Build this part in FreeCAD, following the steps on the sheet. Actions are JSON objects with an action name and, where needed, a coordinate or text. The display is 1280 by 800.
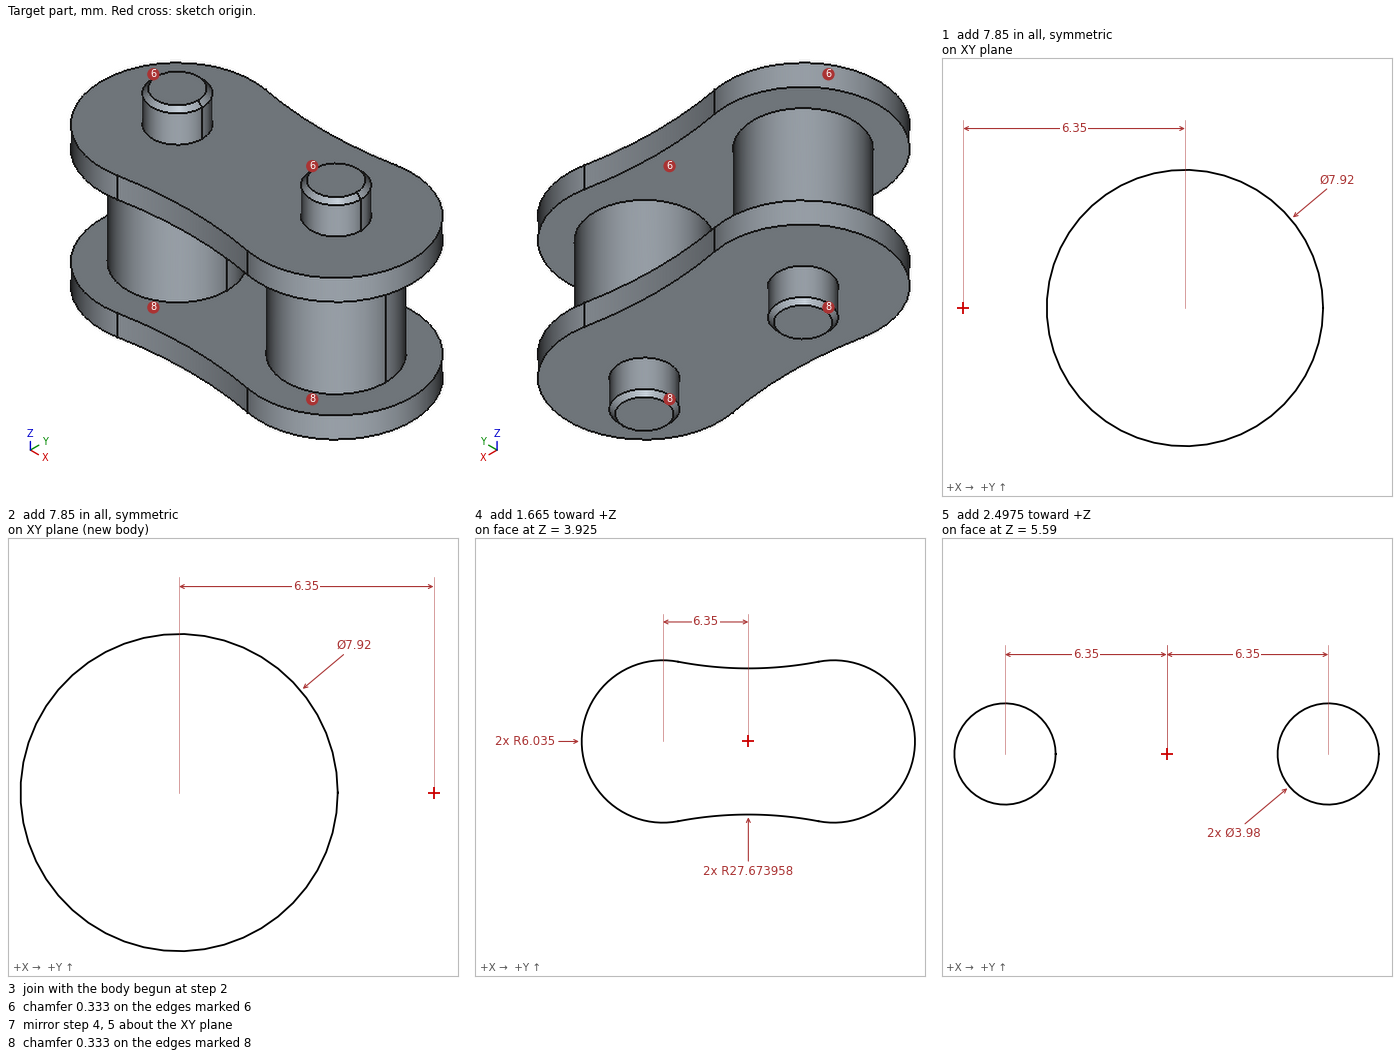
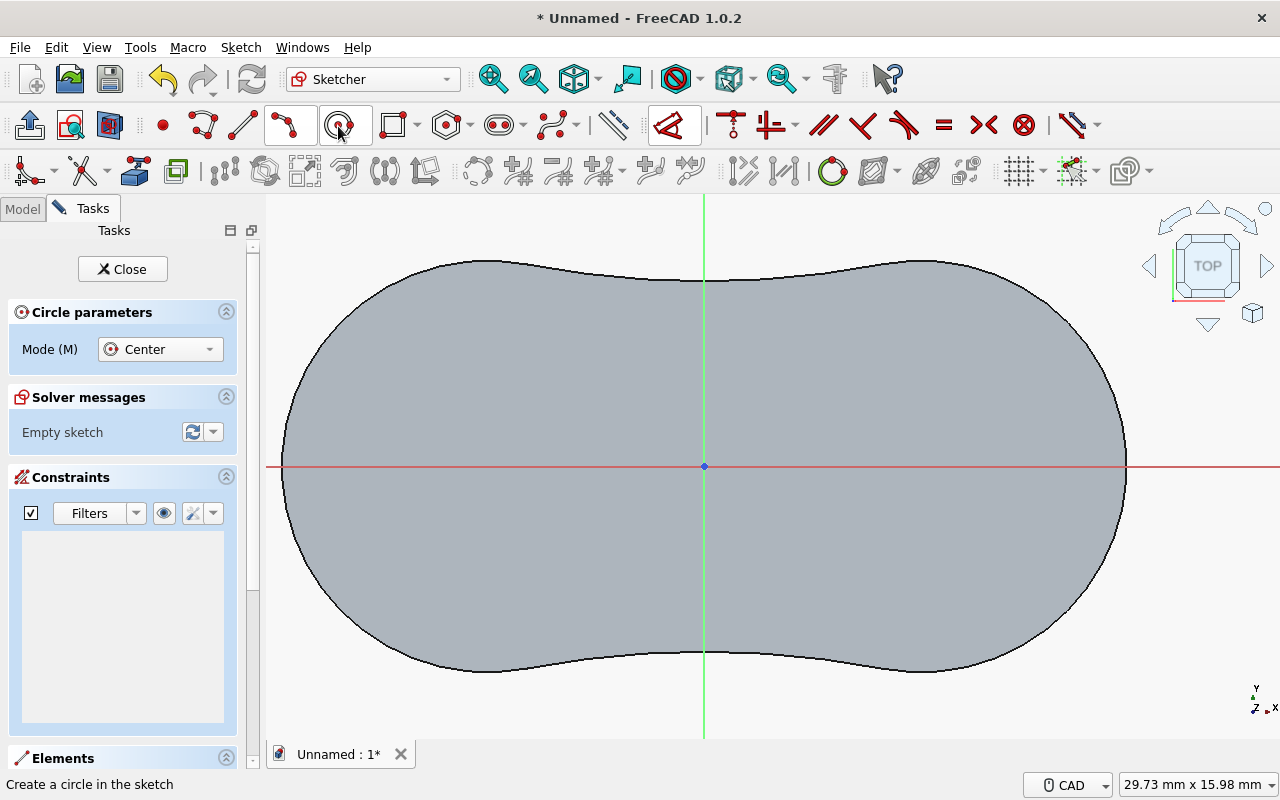
{"action": "left_click", "coordinate": [921, 466]}
{"action": "mouse_move", "coordinate": [969, 419]}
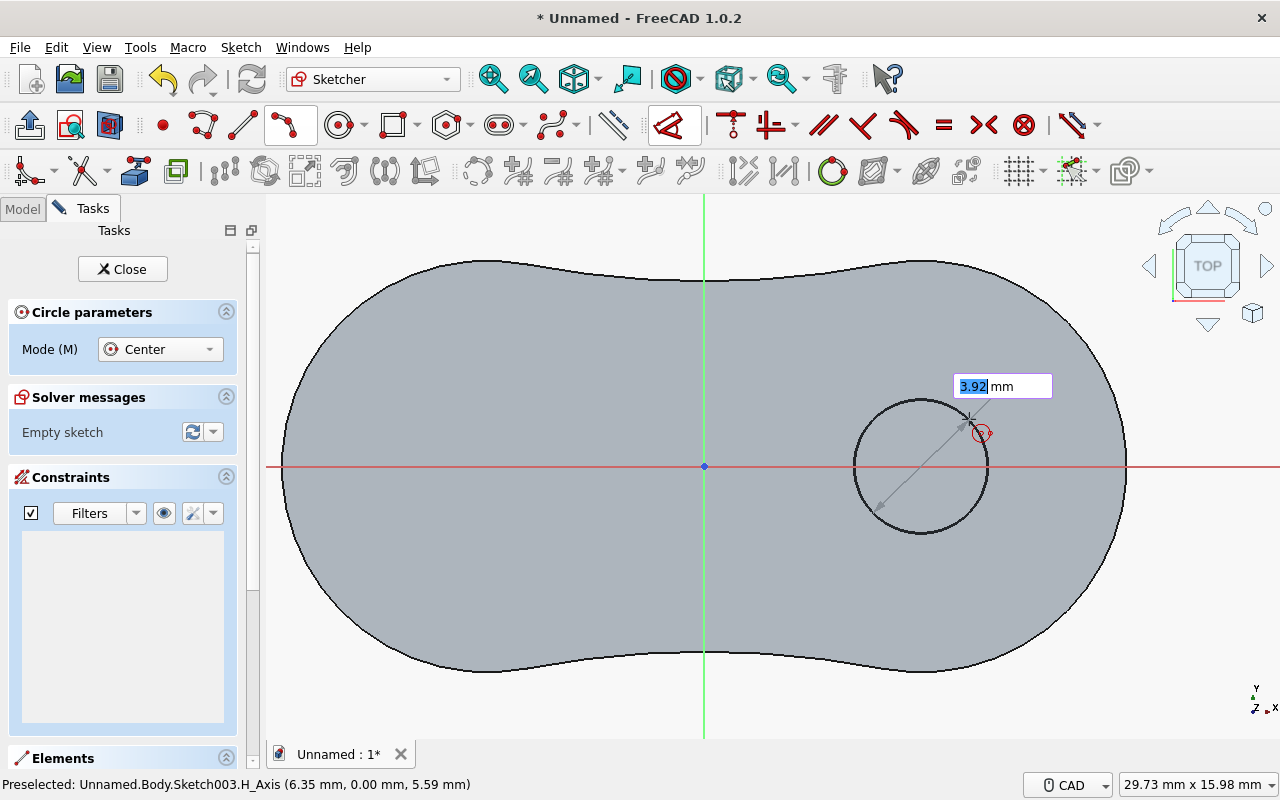
{"action": "type", "text": "3.98"}
{"action": "key", "text": "Return"}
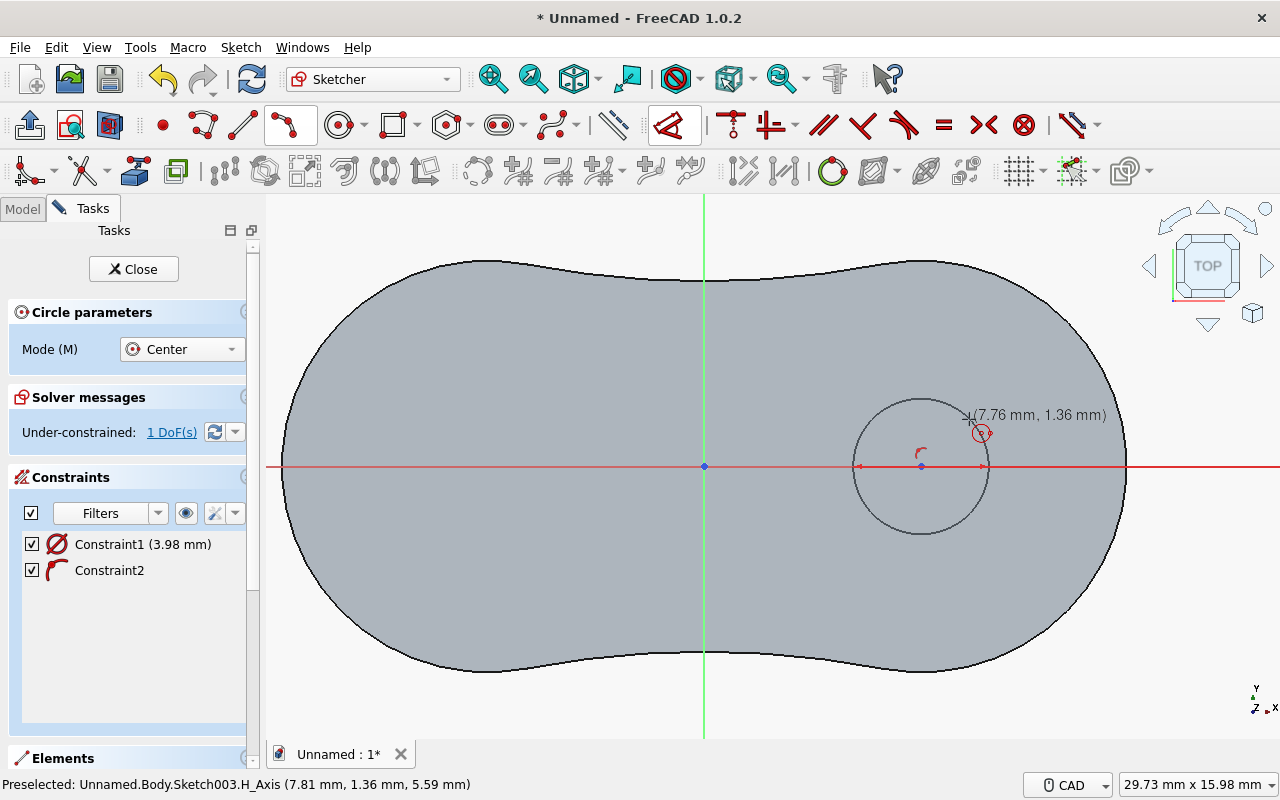
{"action": "left_click", "coordinate": [488, 466]}
{"action": "mouse_move", "coordinate": [536, 419]}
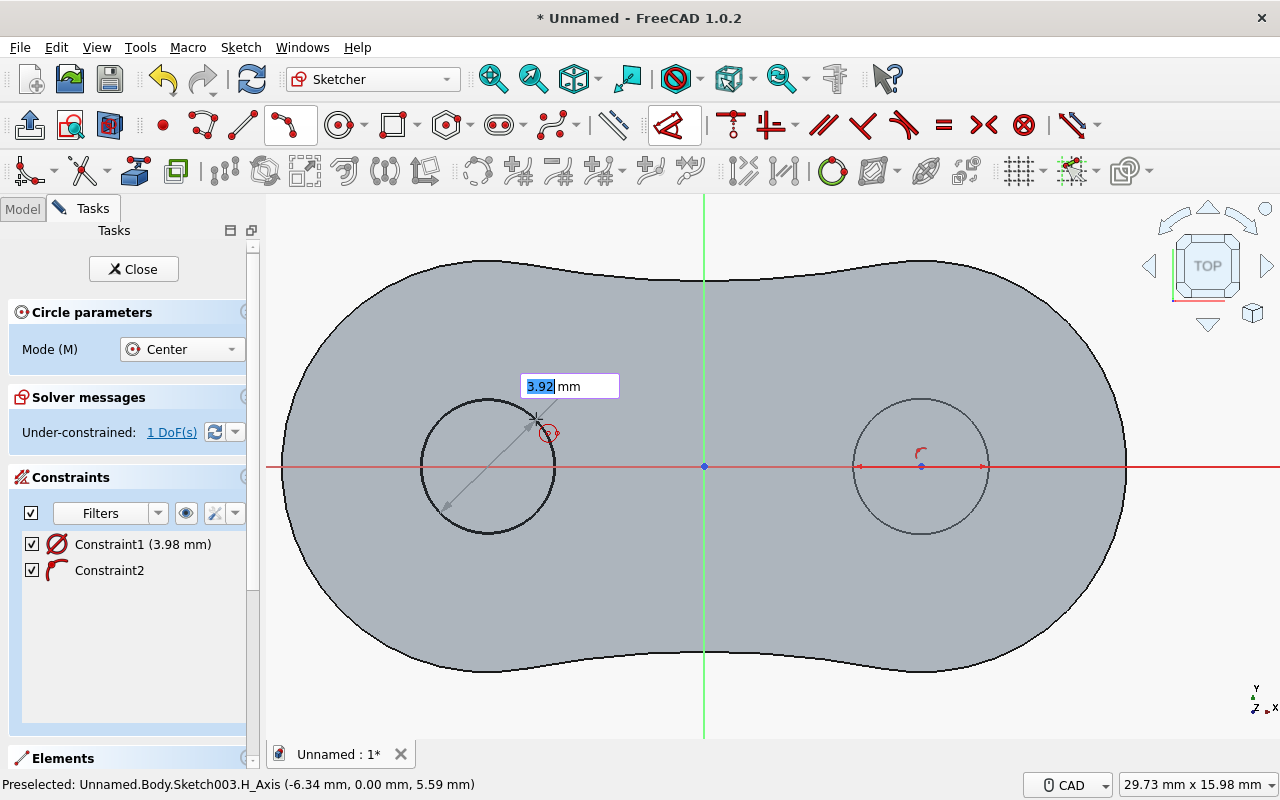
{"action": "type", "text": "3.98"}
{"action": "key", "text": "Return"}
{"action": "key", "text": "Escape"}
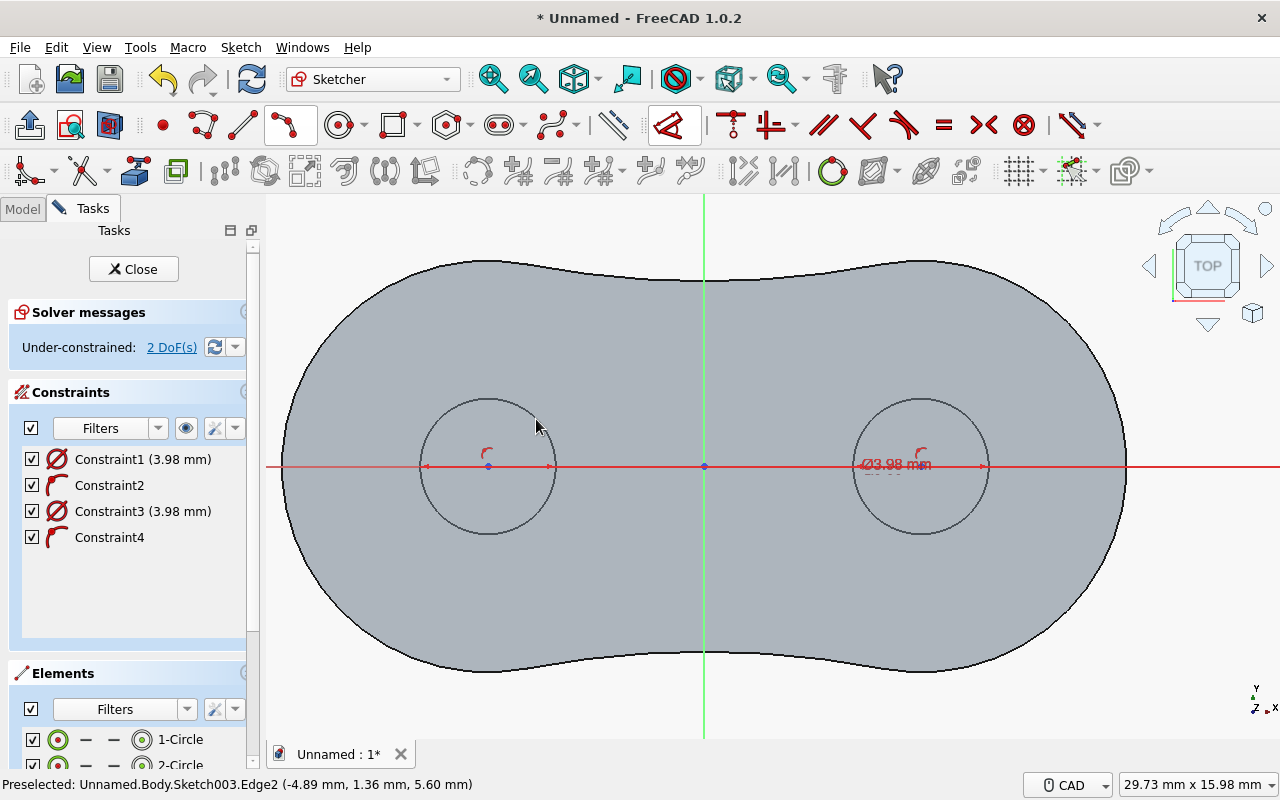
{"action": "left_click", "coordinate": [921, 466]}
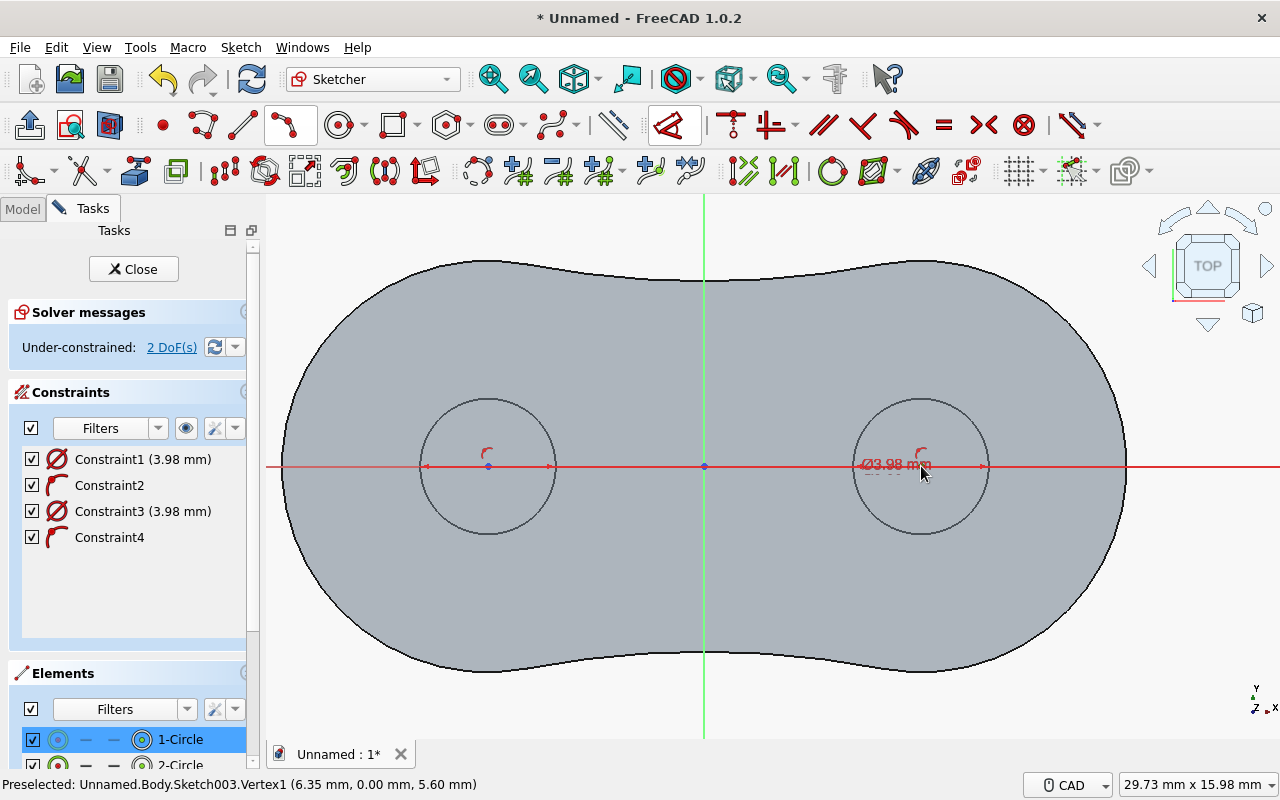
{"action": "left_click", "coordinate": [696, 126]}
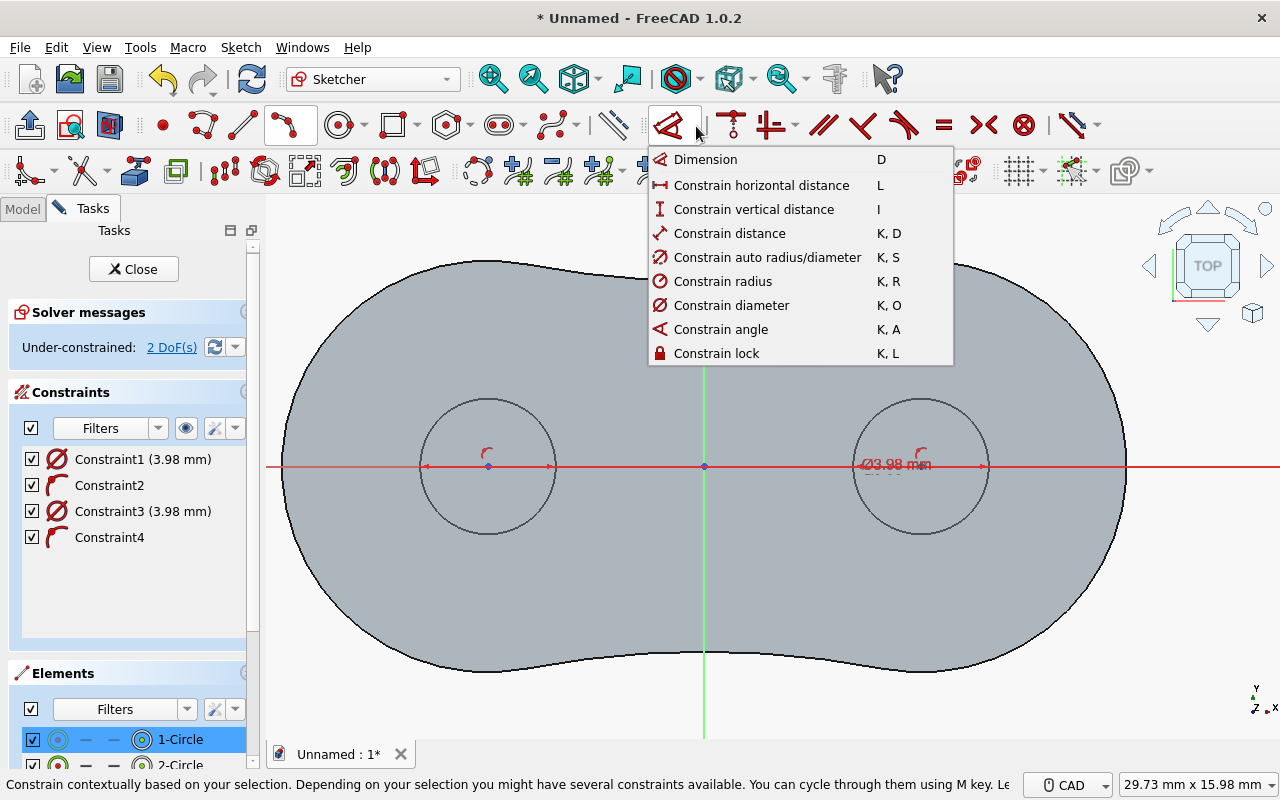
{"action": "left_click", "coordinate": [801, 185]}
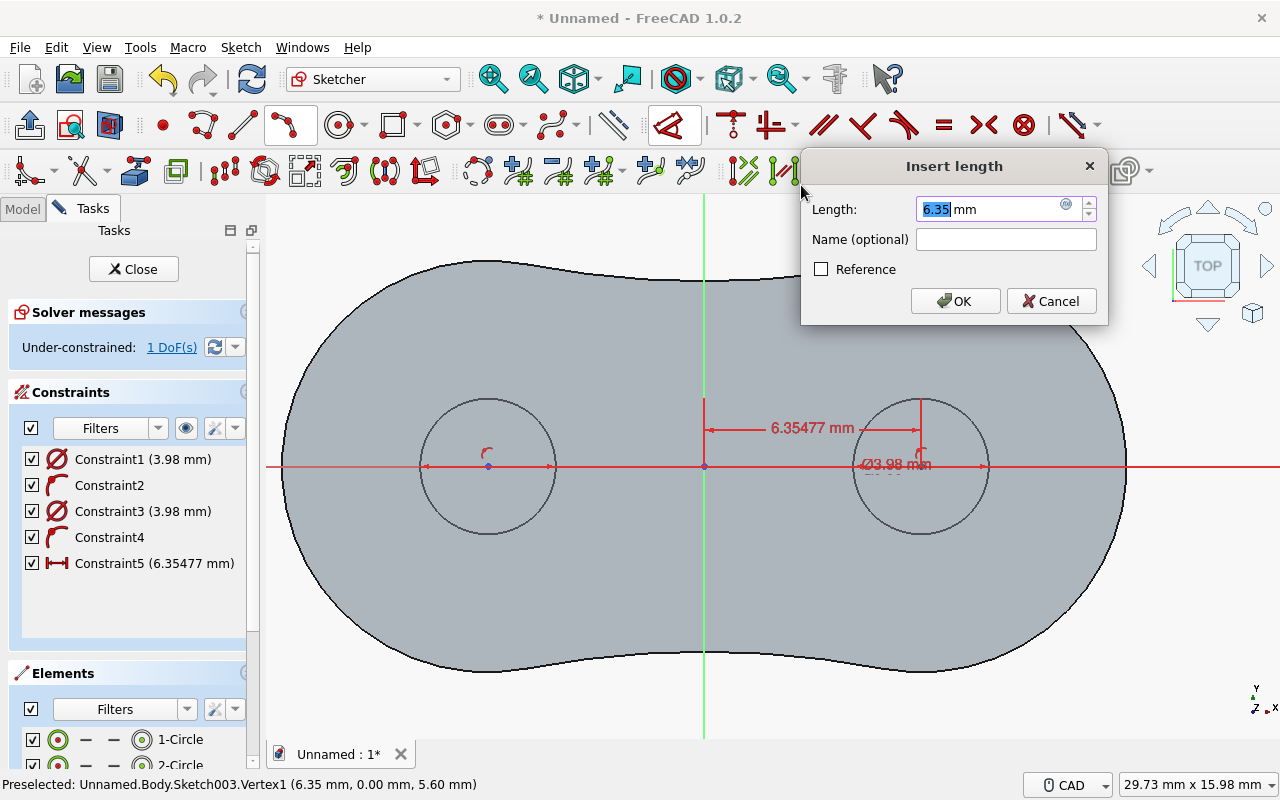
{"action": "type", "text": "6.35"}
{"action": "key", "text": "Return"}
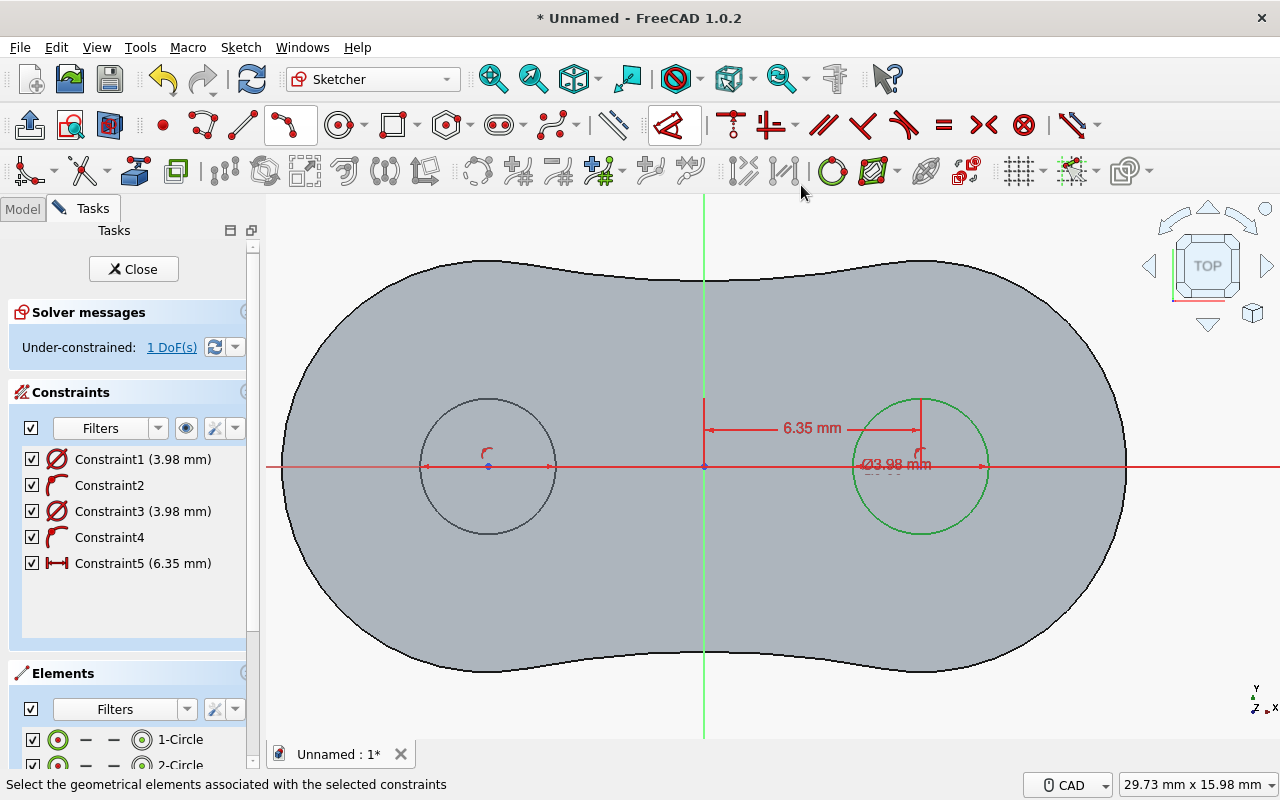
{"action": "left_click", "coordinate": [488, 466]}